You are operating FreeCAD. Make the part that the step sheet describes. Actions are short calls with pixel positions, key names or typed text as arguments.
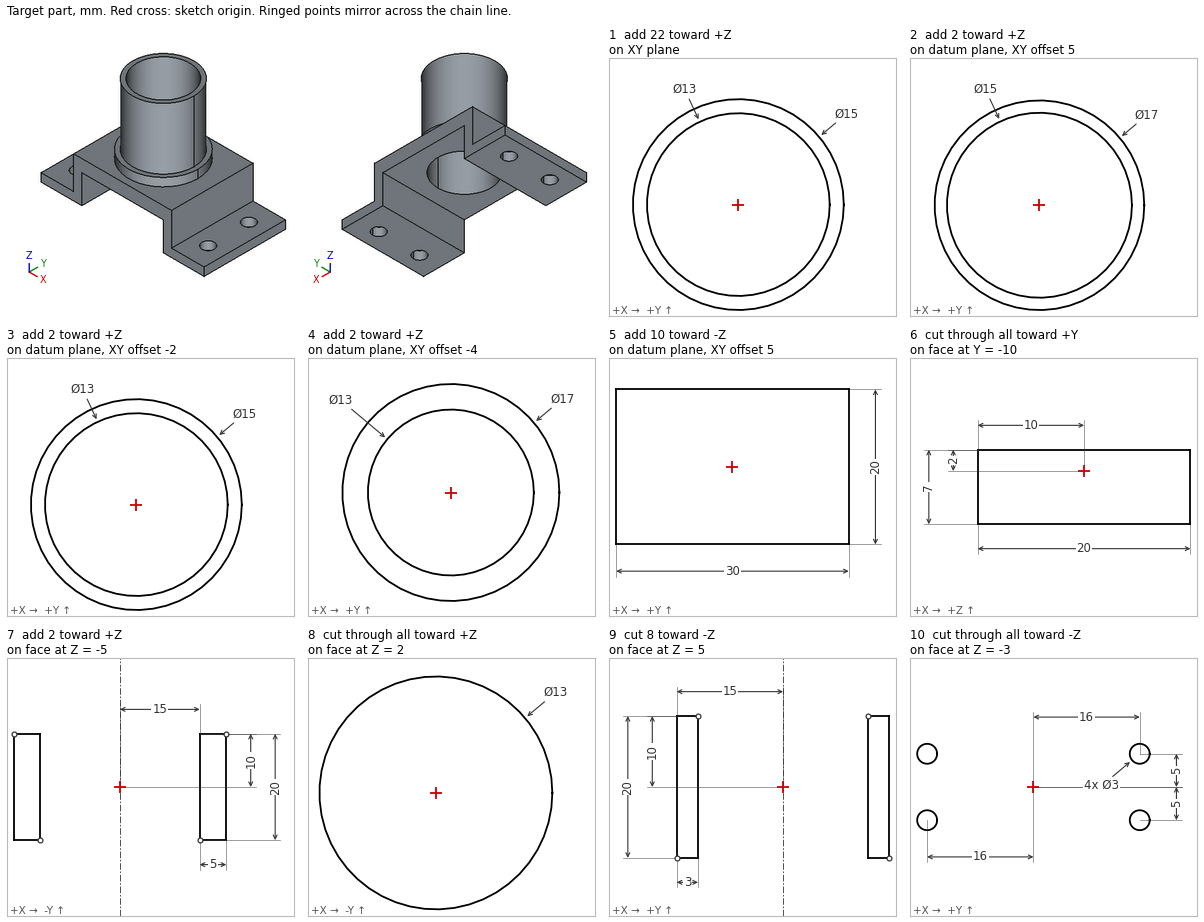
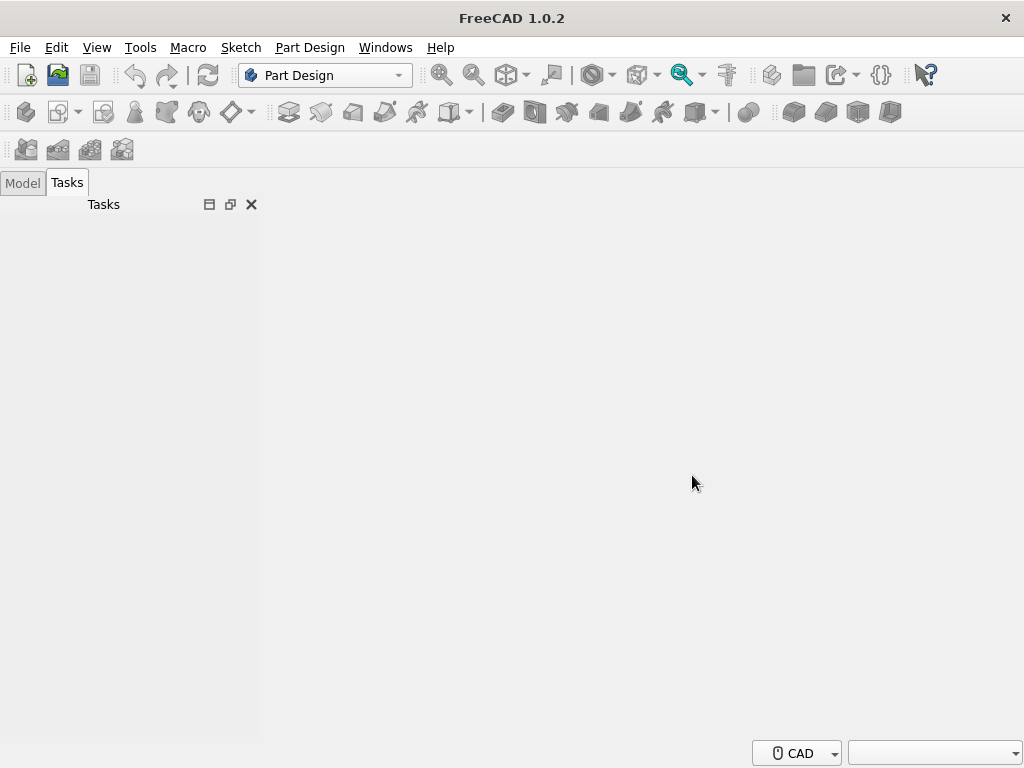
click(26, 76)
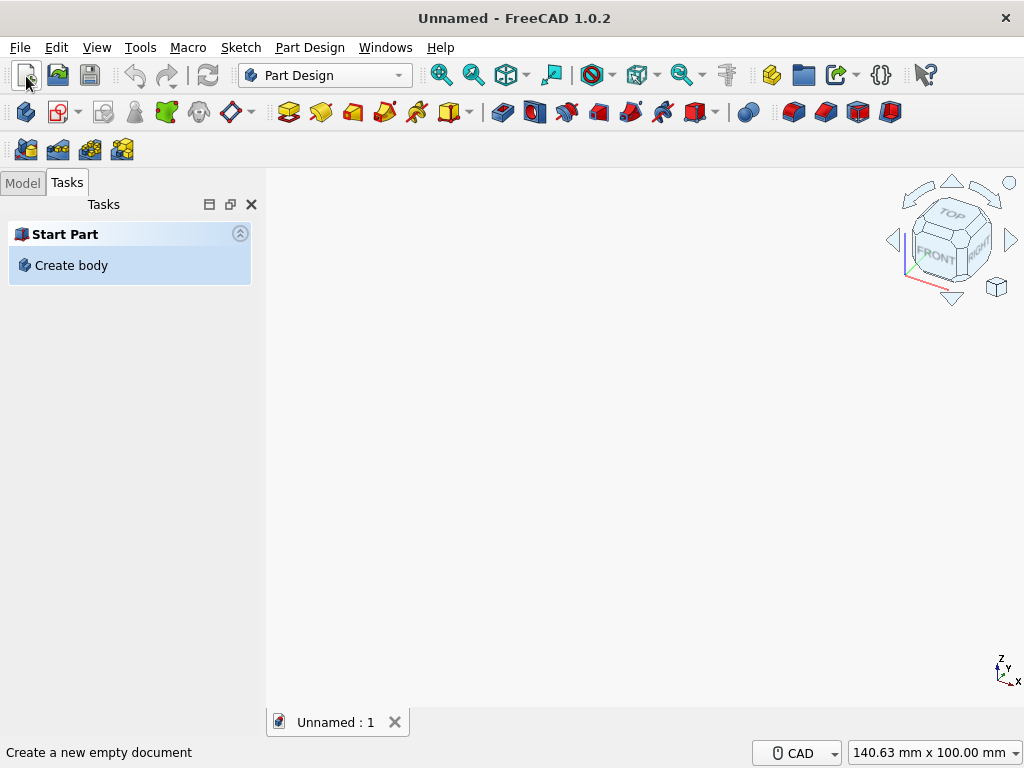
click(58, 112)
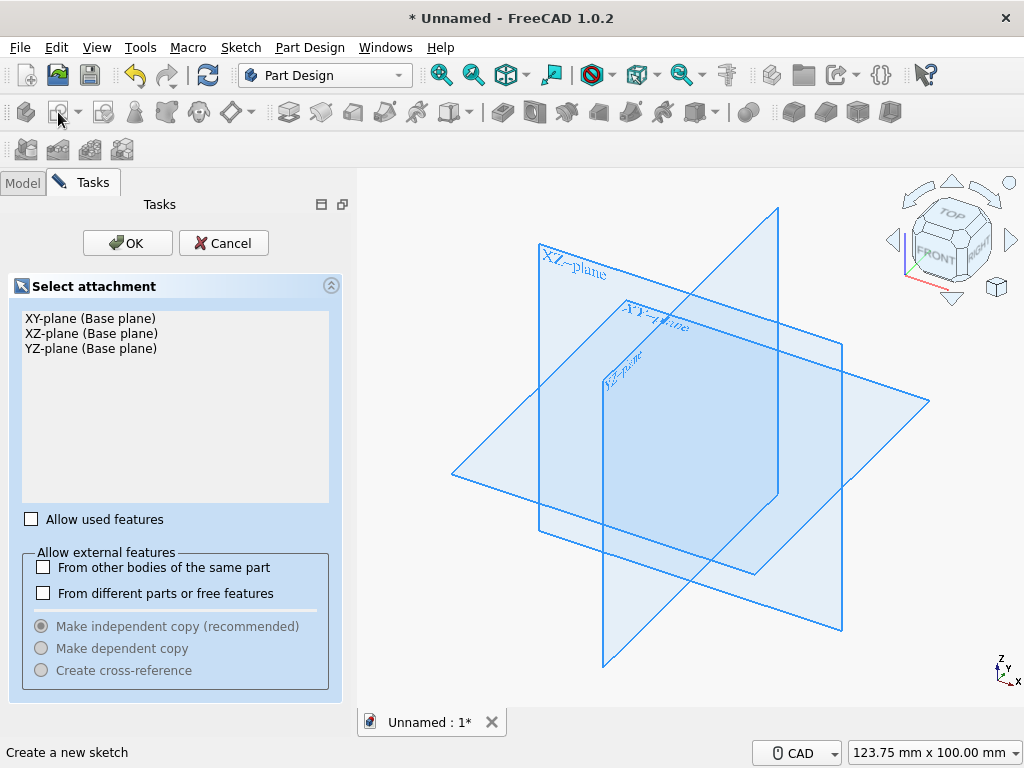
click(82, 318)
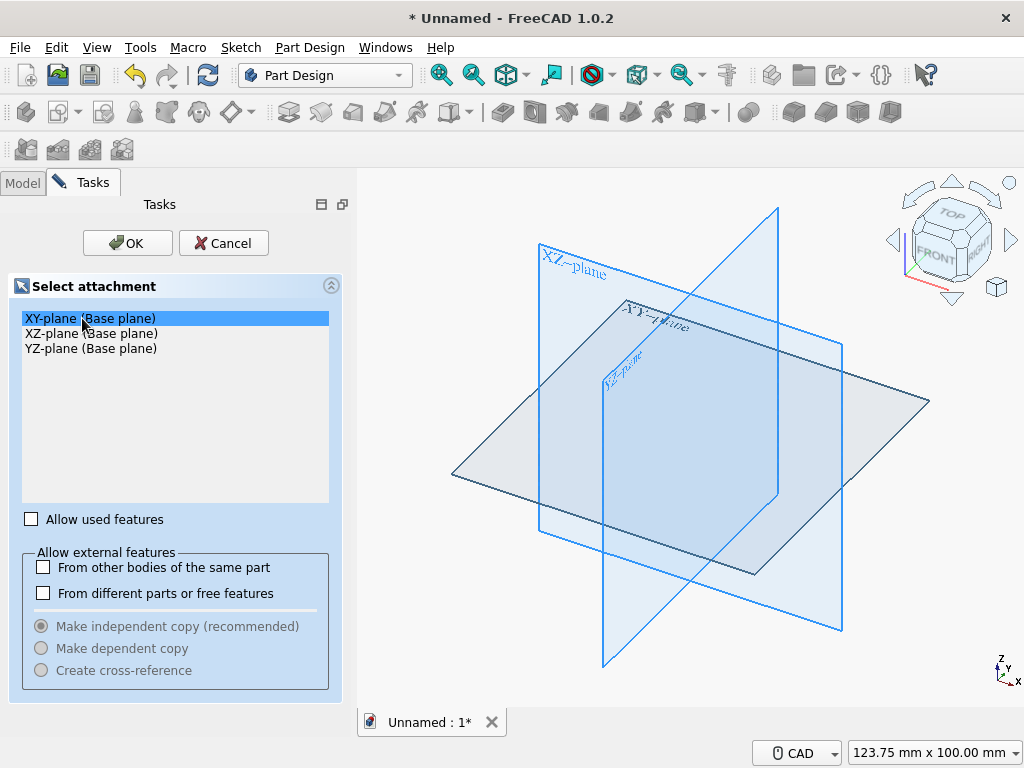
click(128, 243)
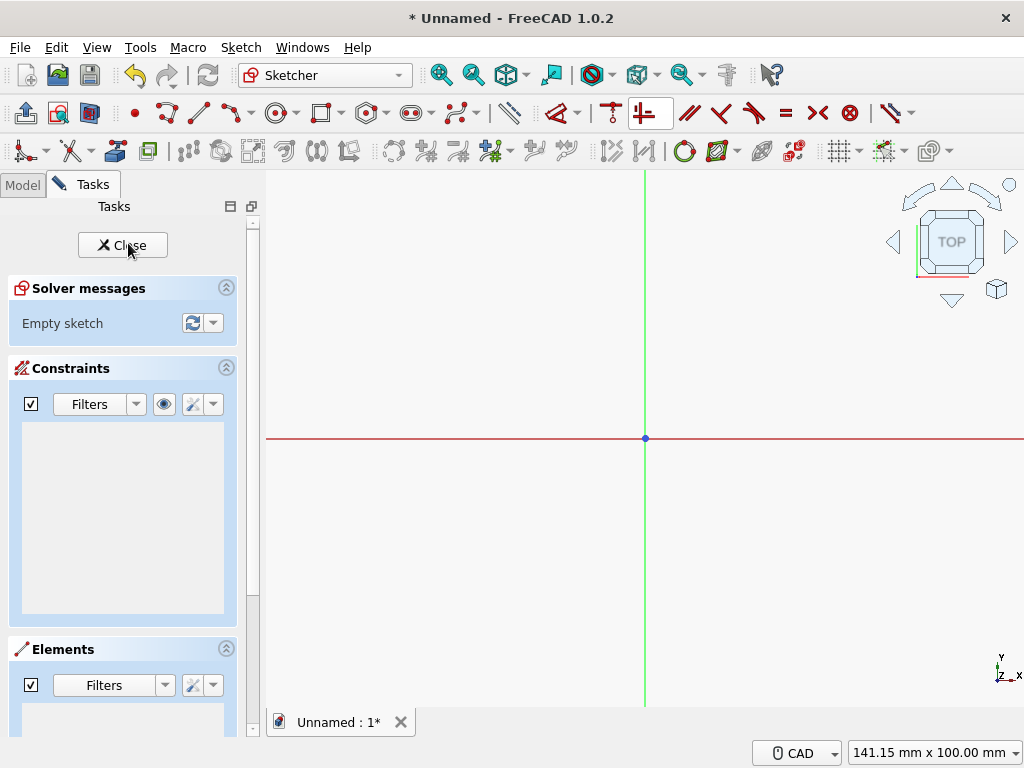
scroll(667, 438, up, 7)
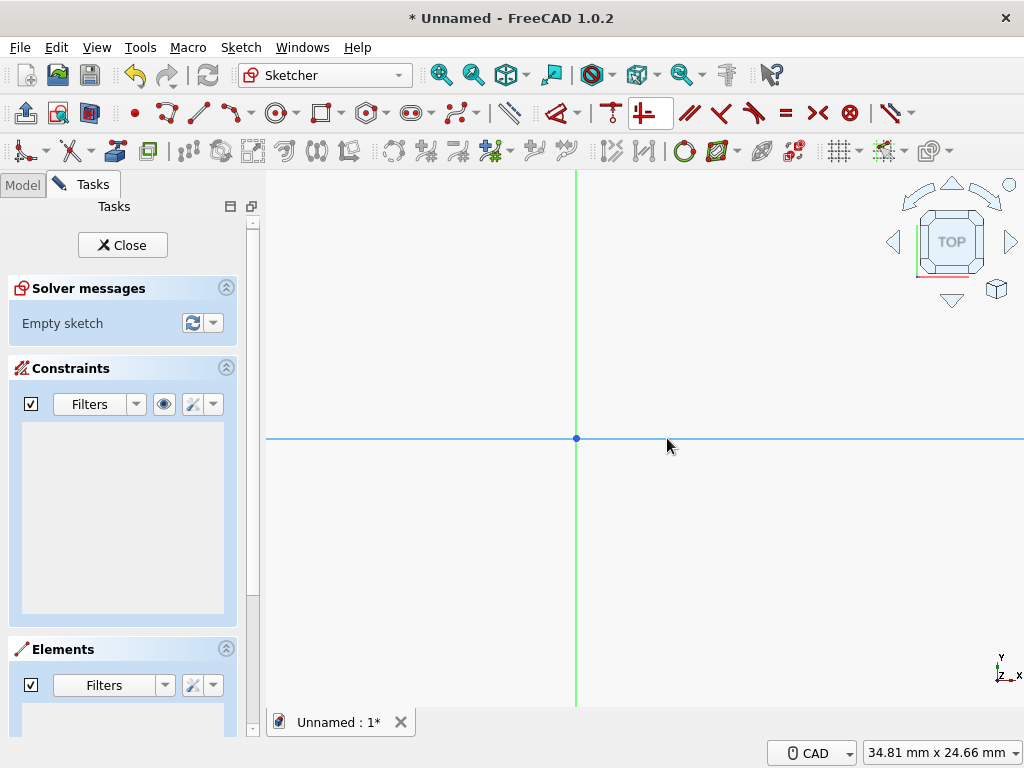
click(276, 114)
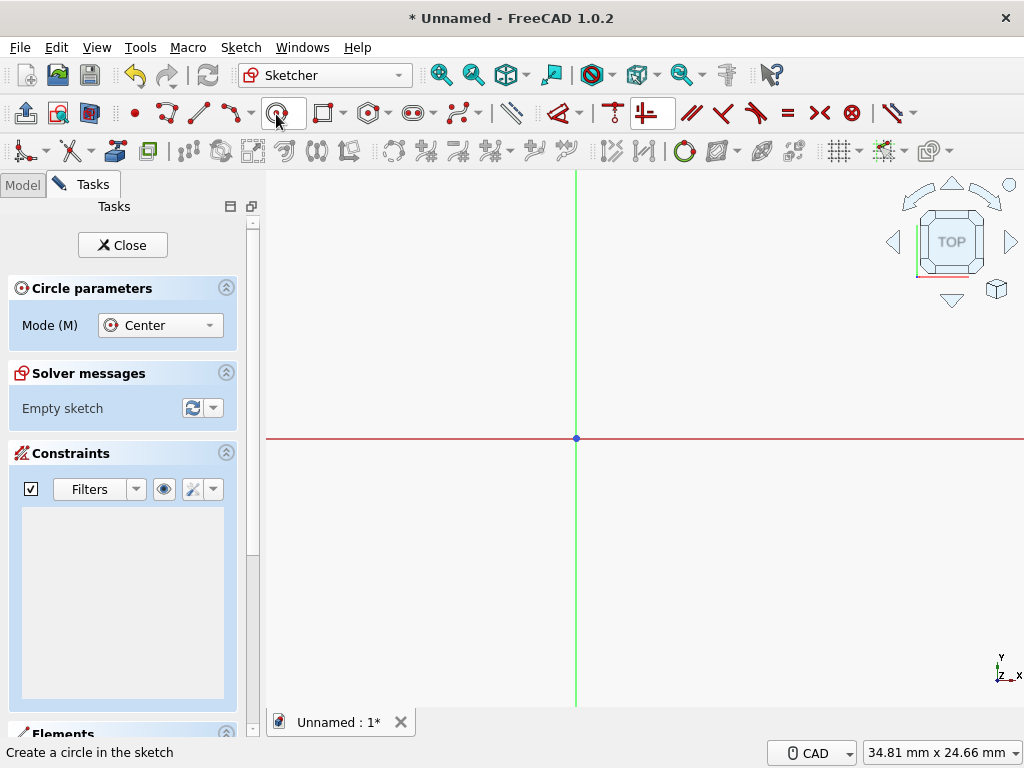
click(576, 438)
click(692, 323)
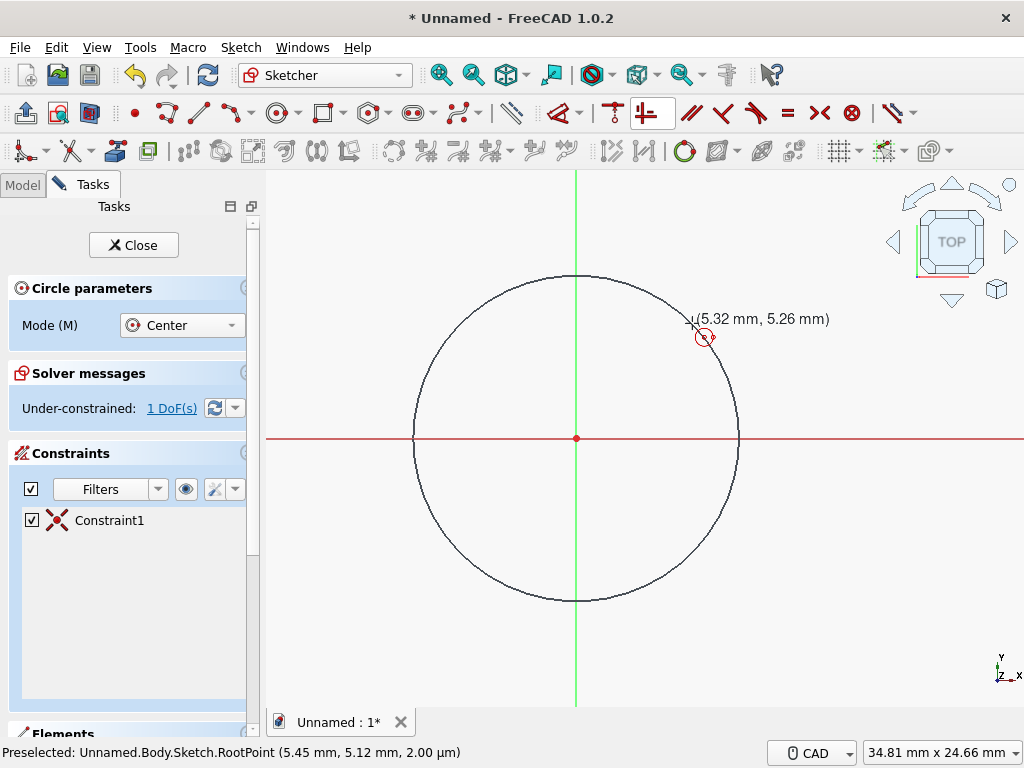
click(576, 438)
click(676, 338)
key(Escape)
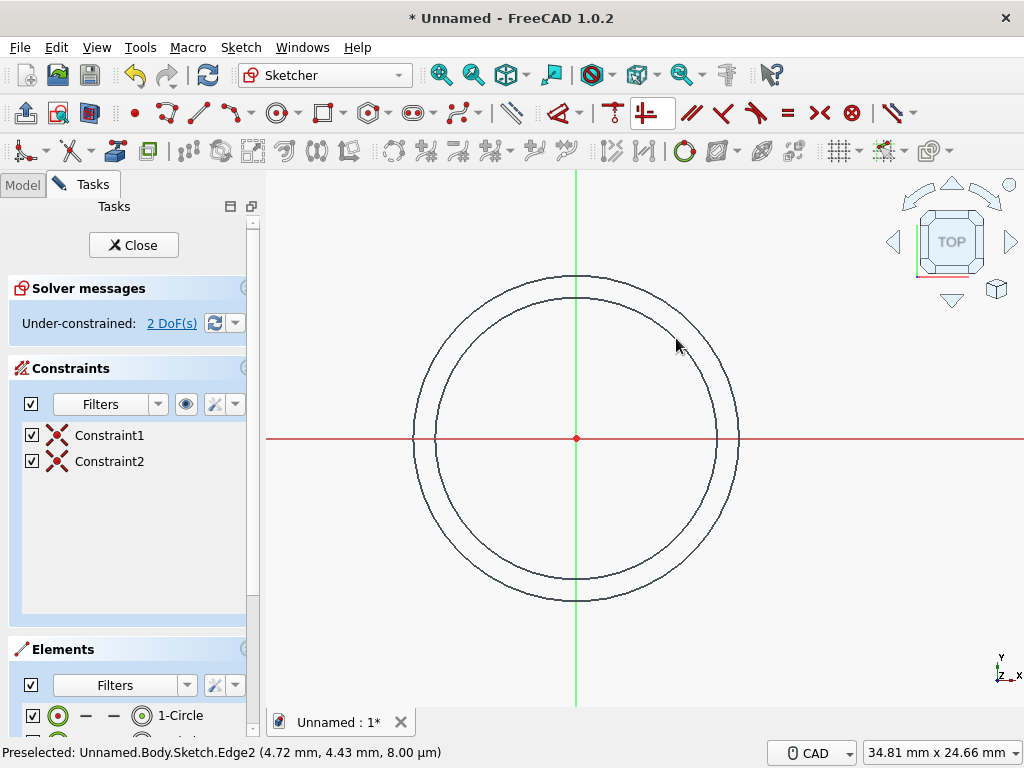
click(558, 114)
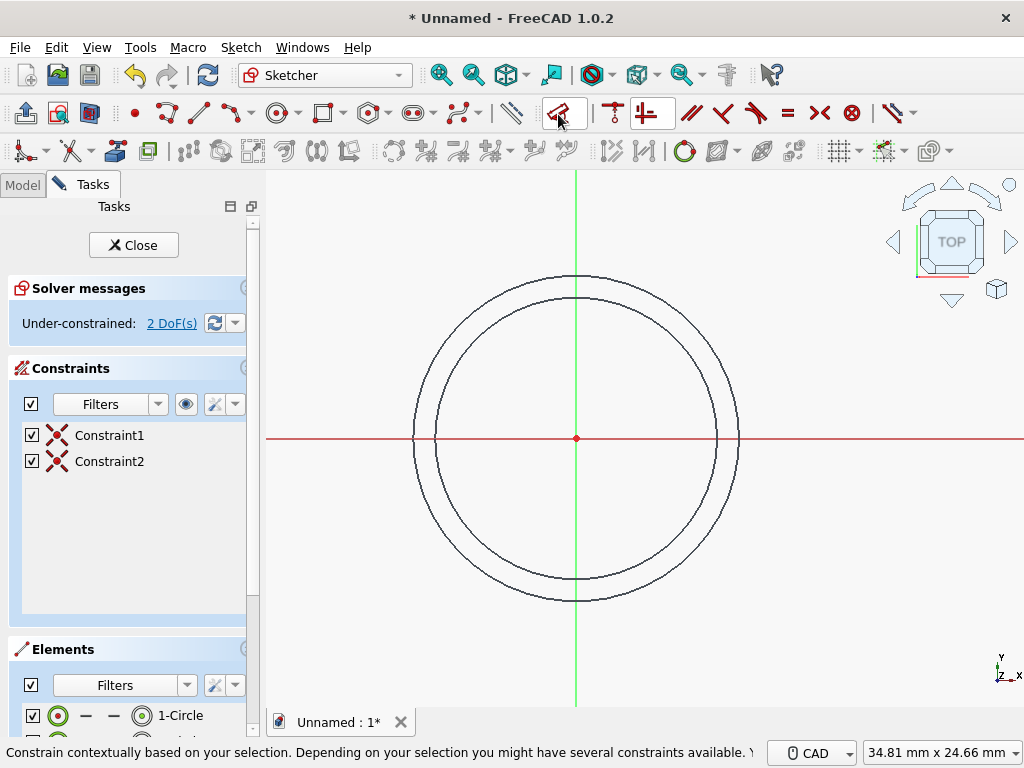
click(691, 323)
click(714, 300)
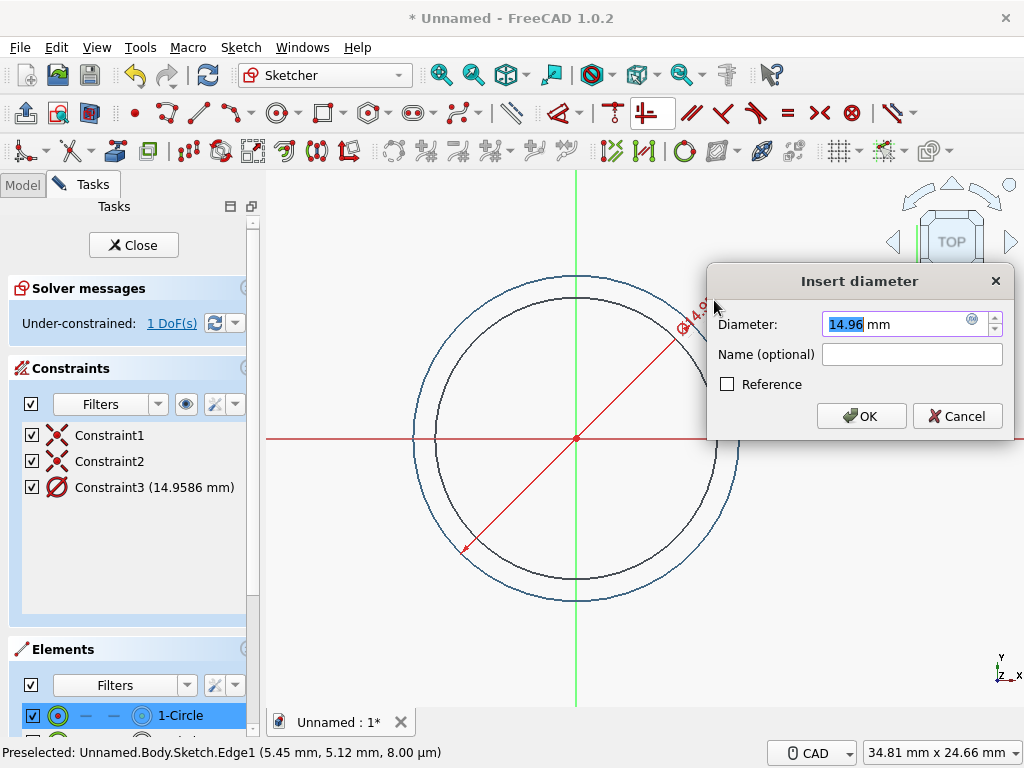
text(15)
key(Return)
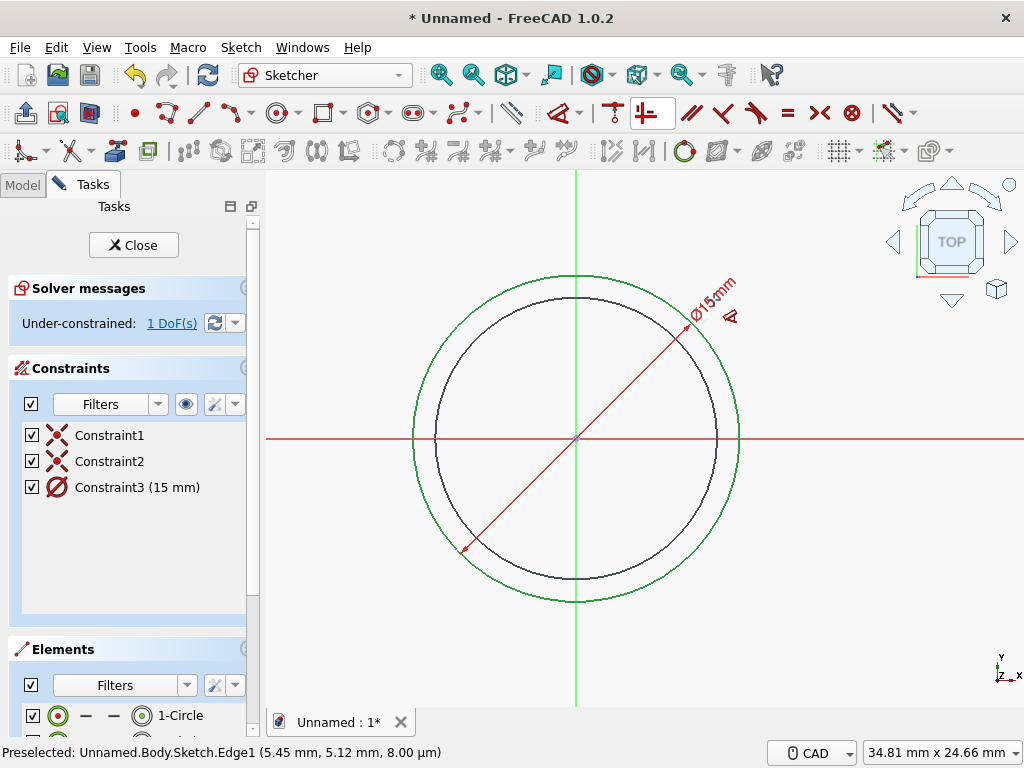
click(676, 339)
click(764, 384)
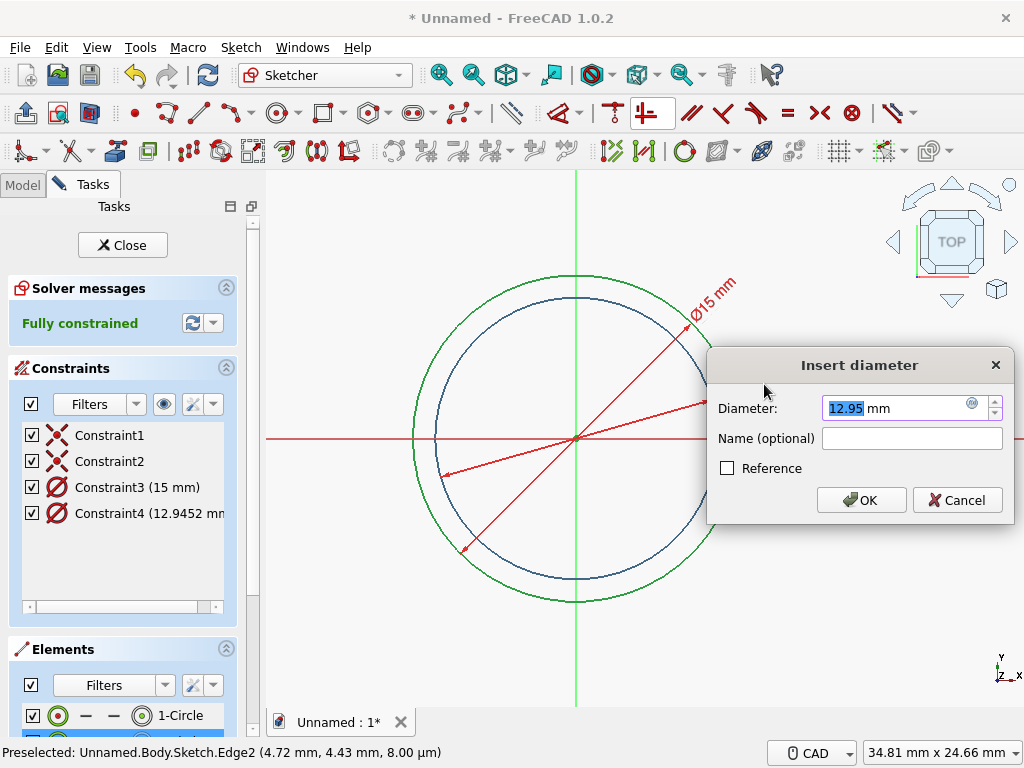
text(13)
key(Return)
key(Escape)